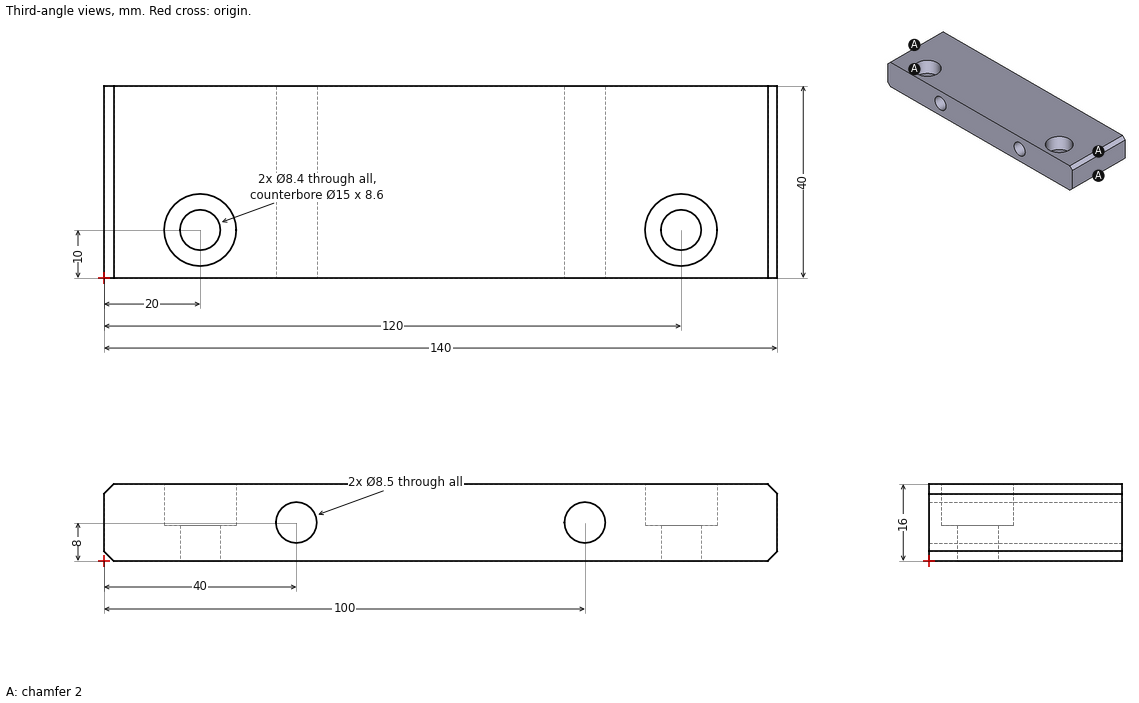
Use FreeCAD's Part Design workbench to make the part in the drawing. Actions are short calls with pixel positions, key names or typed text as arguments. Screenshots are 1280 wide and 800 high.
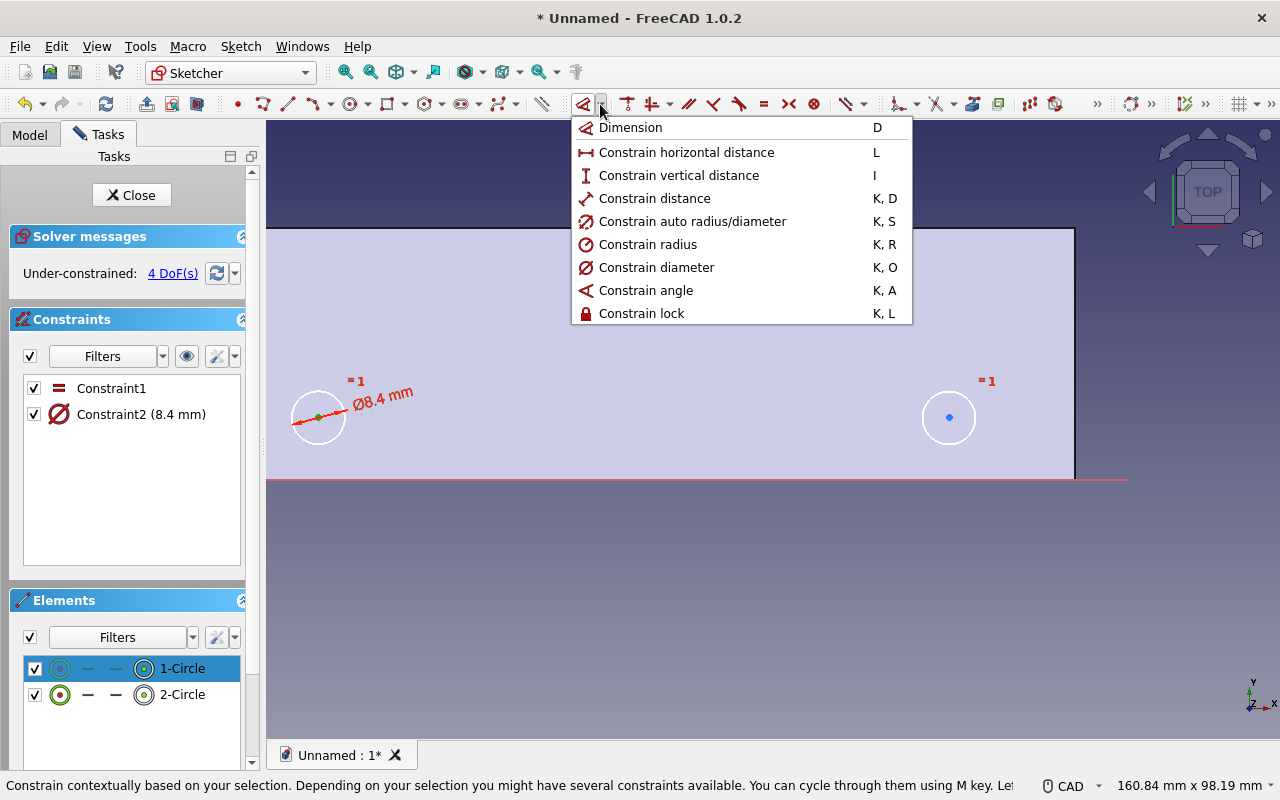
click(742, 152)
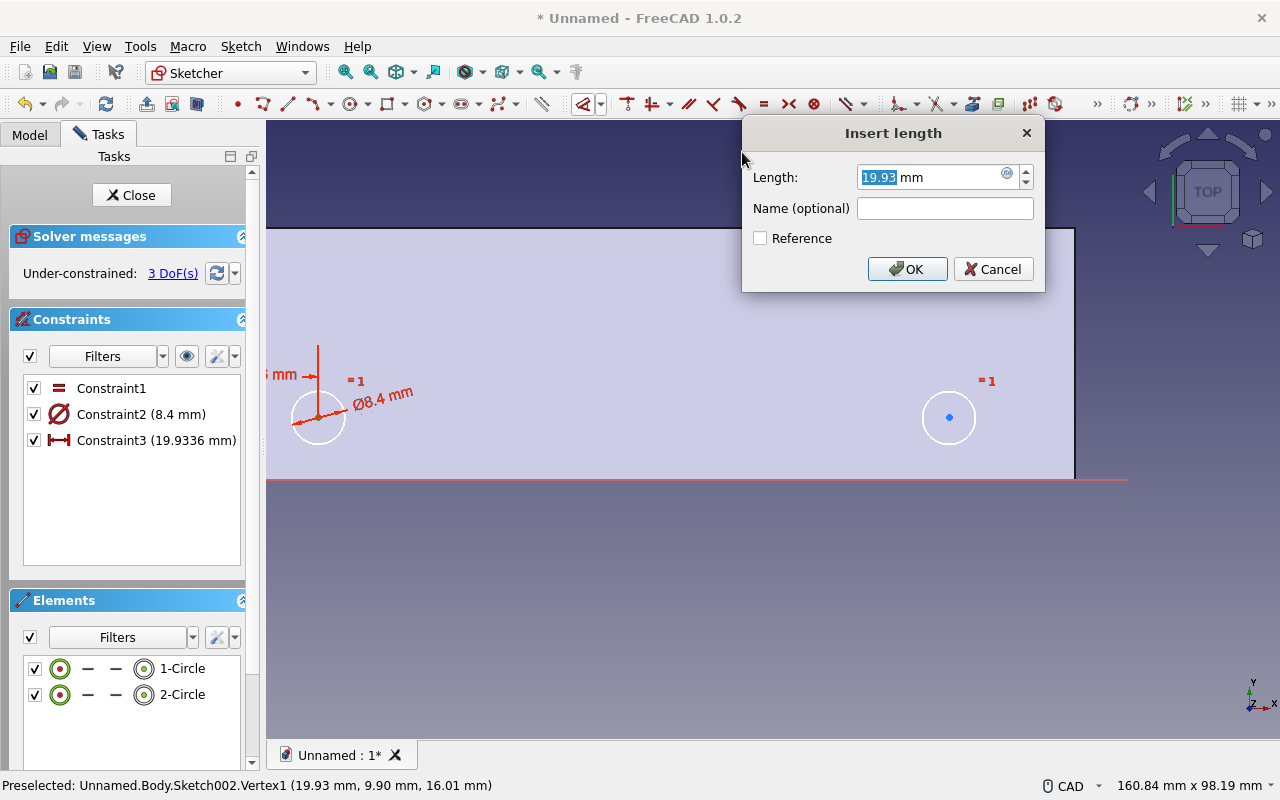
text(20)
key(Return)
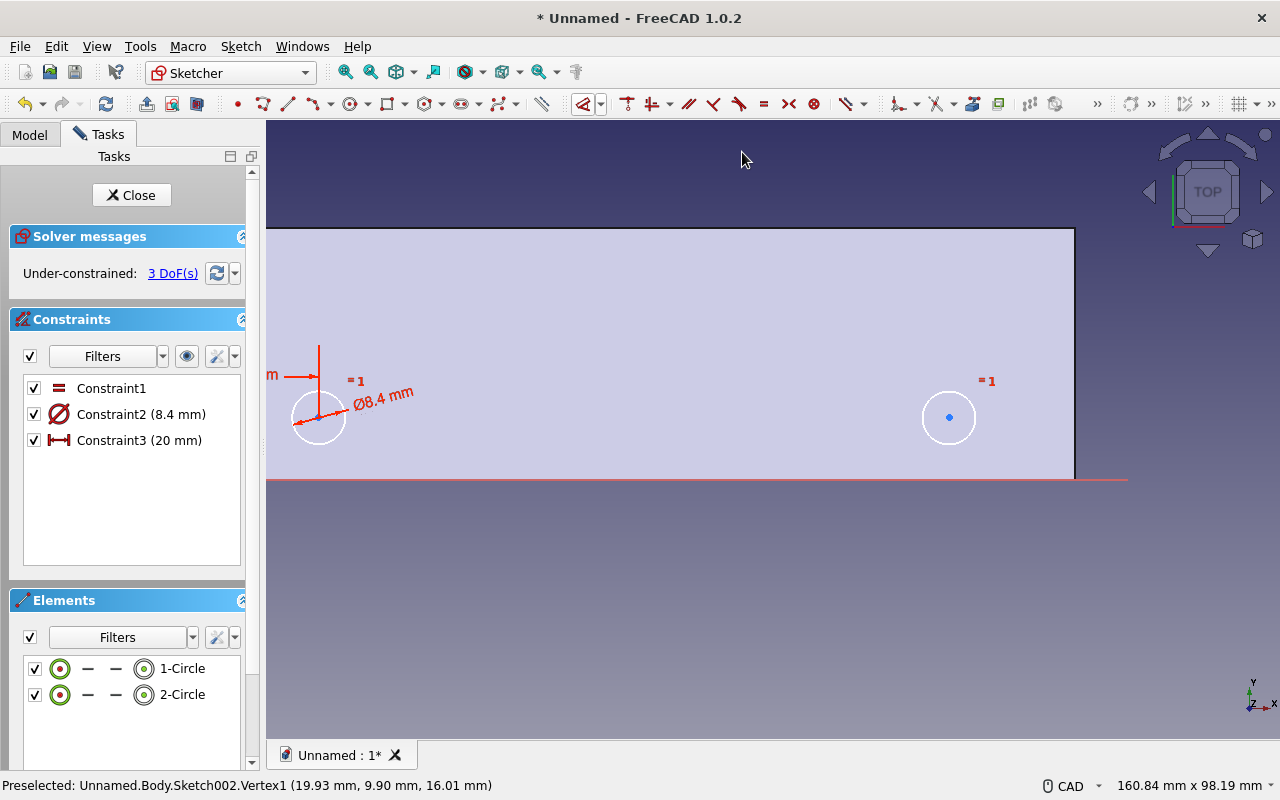
click(319, 418)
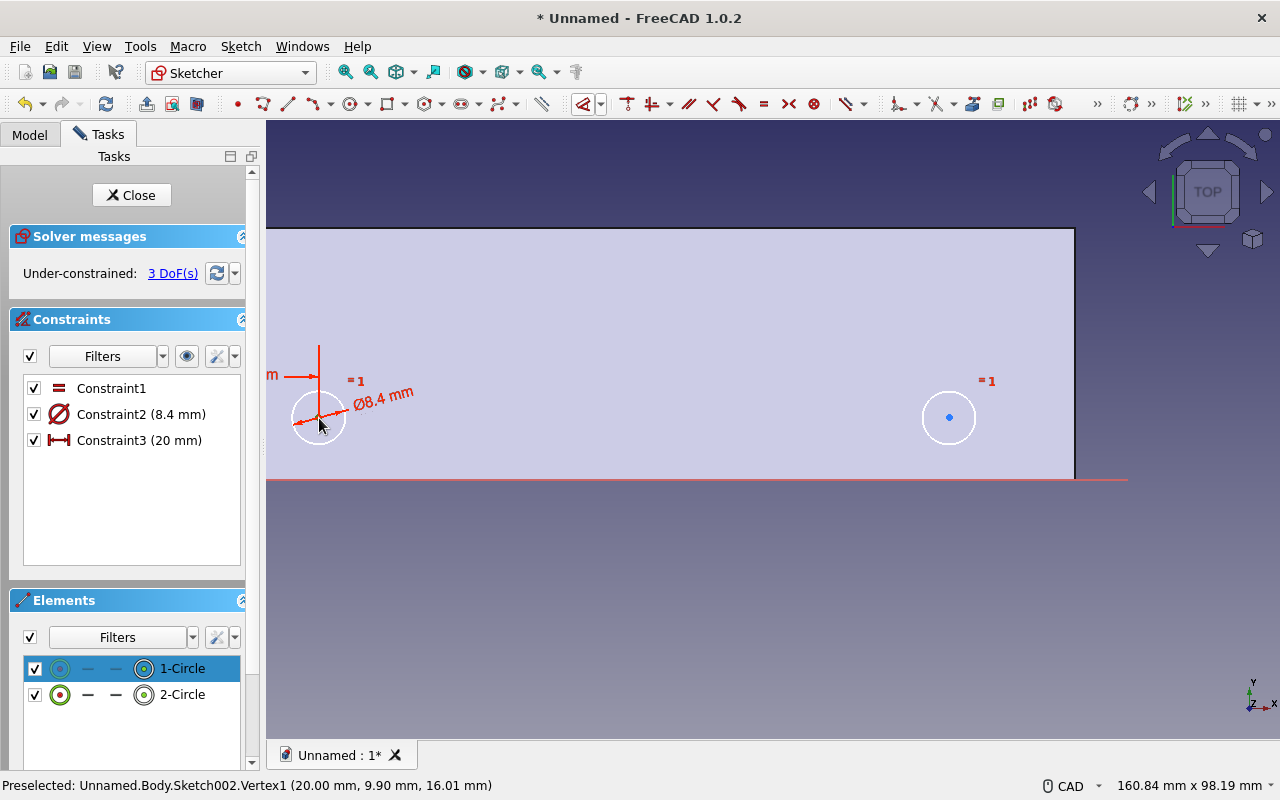
key(i)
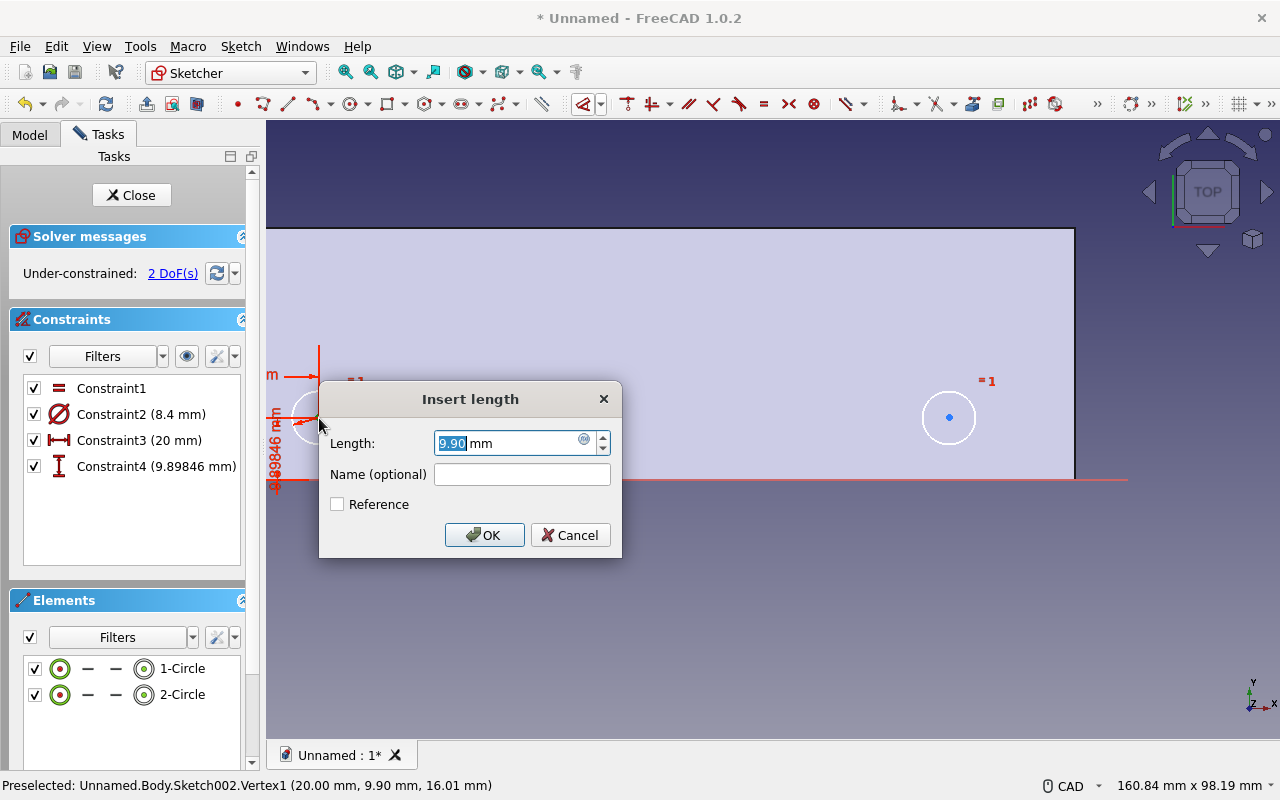
text(10)
key(Return)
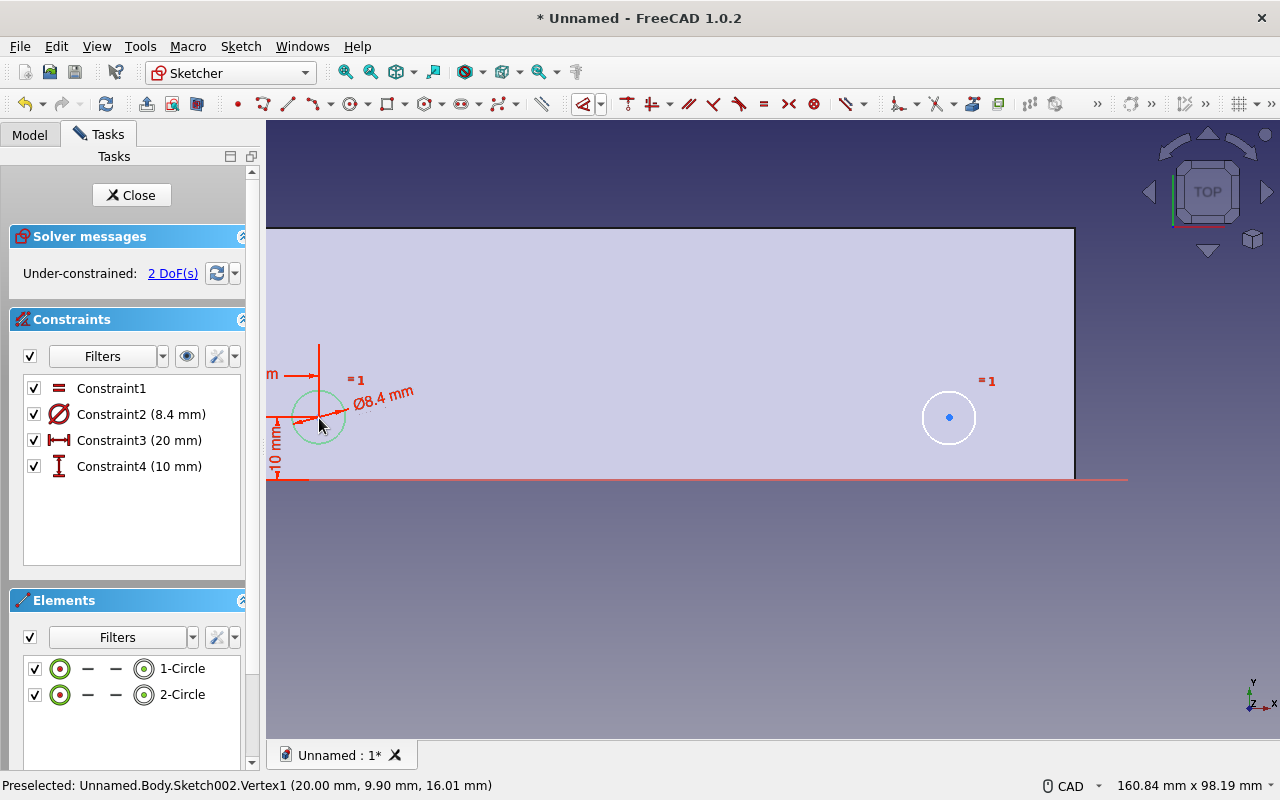
click(949, 418)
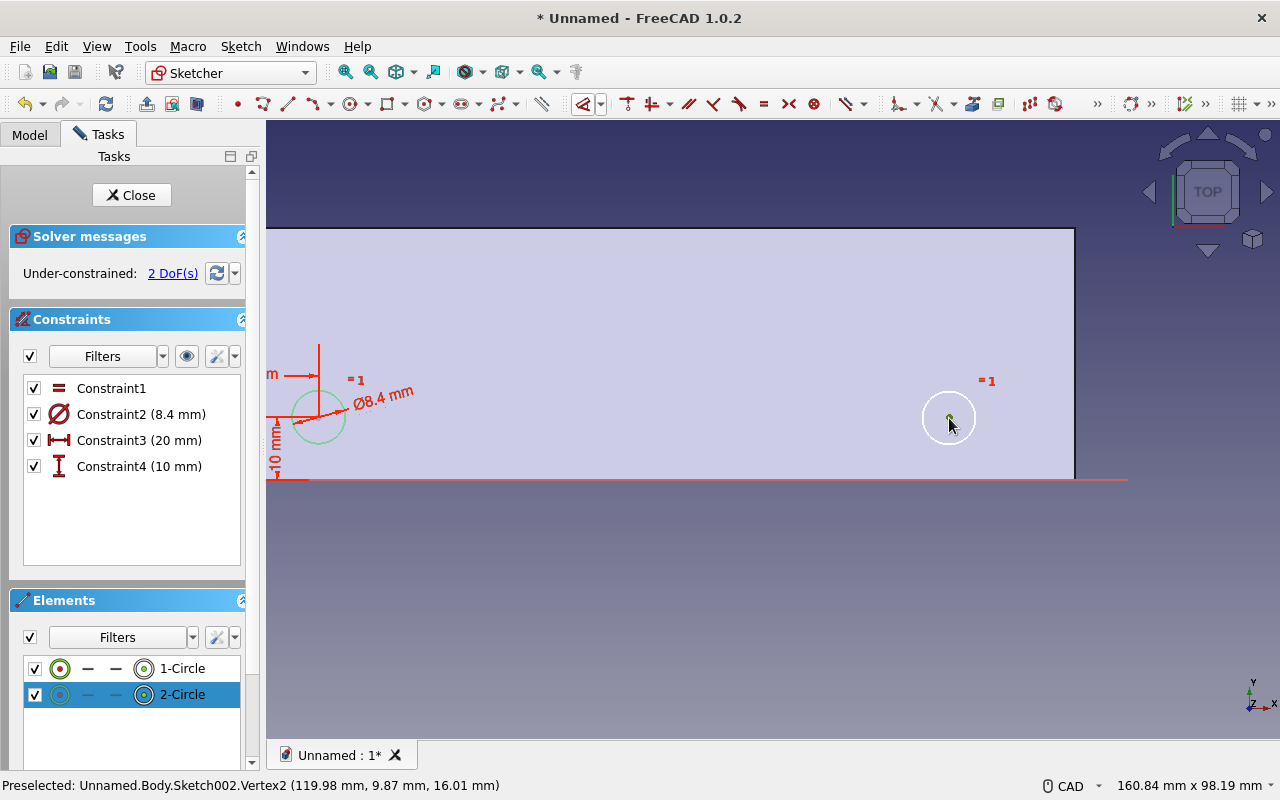
click(600, 104)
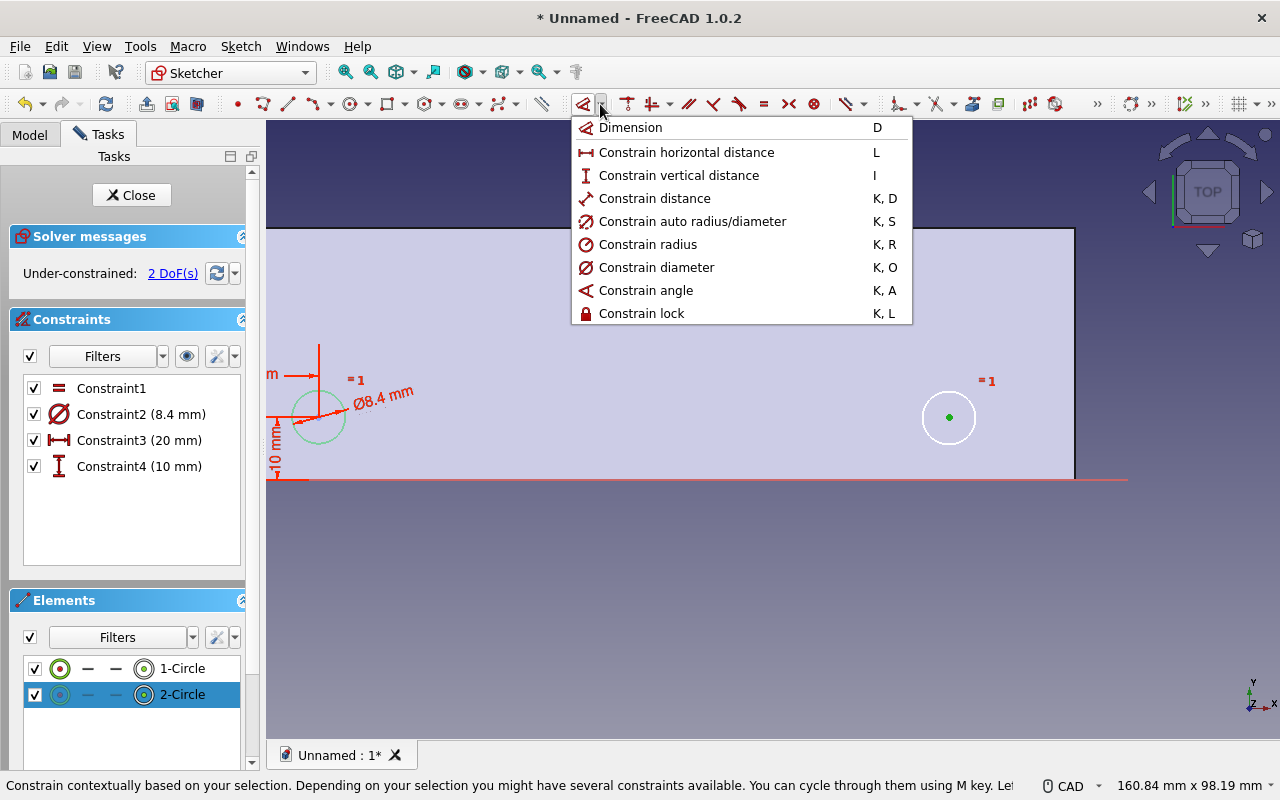
click(742, 176)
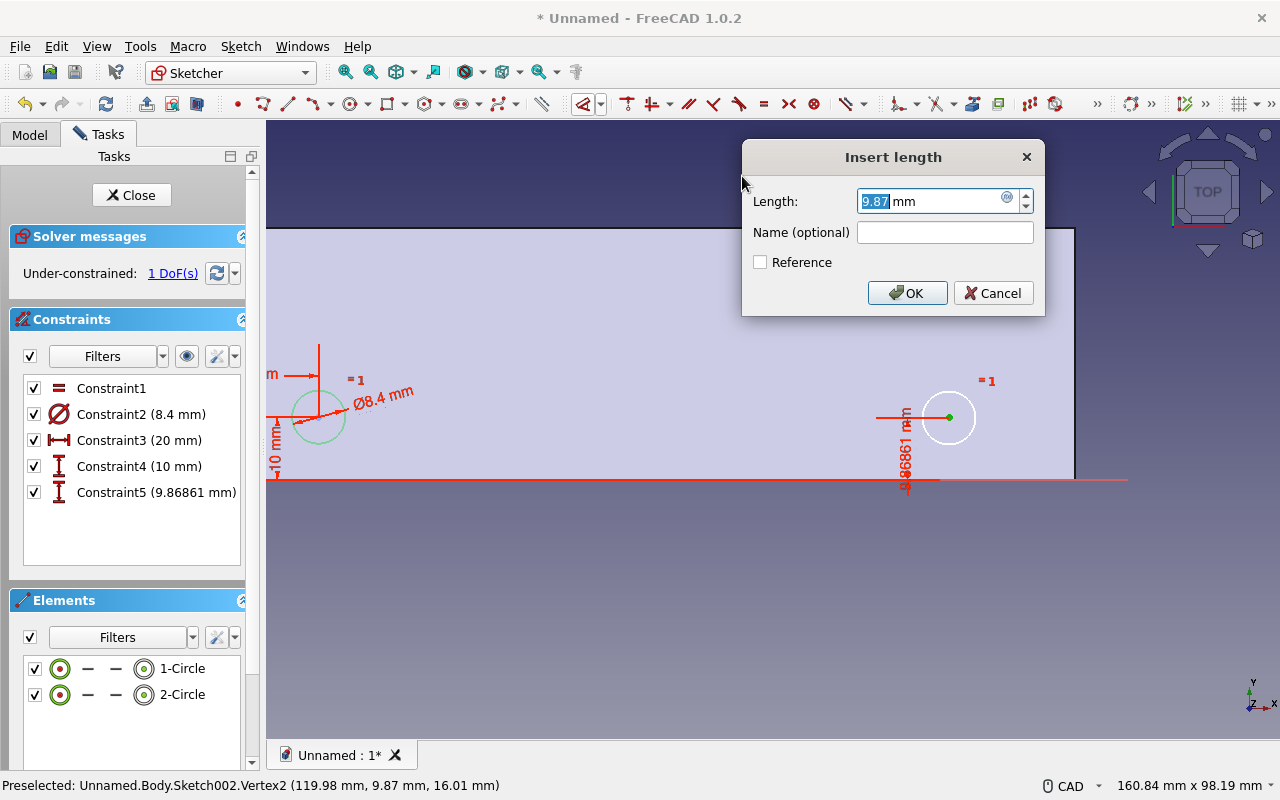
text(10)
key(Return)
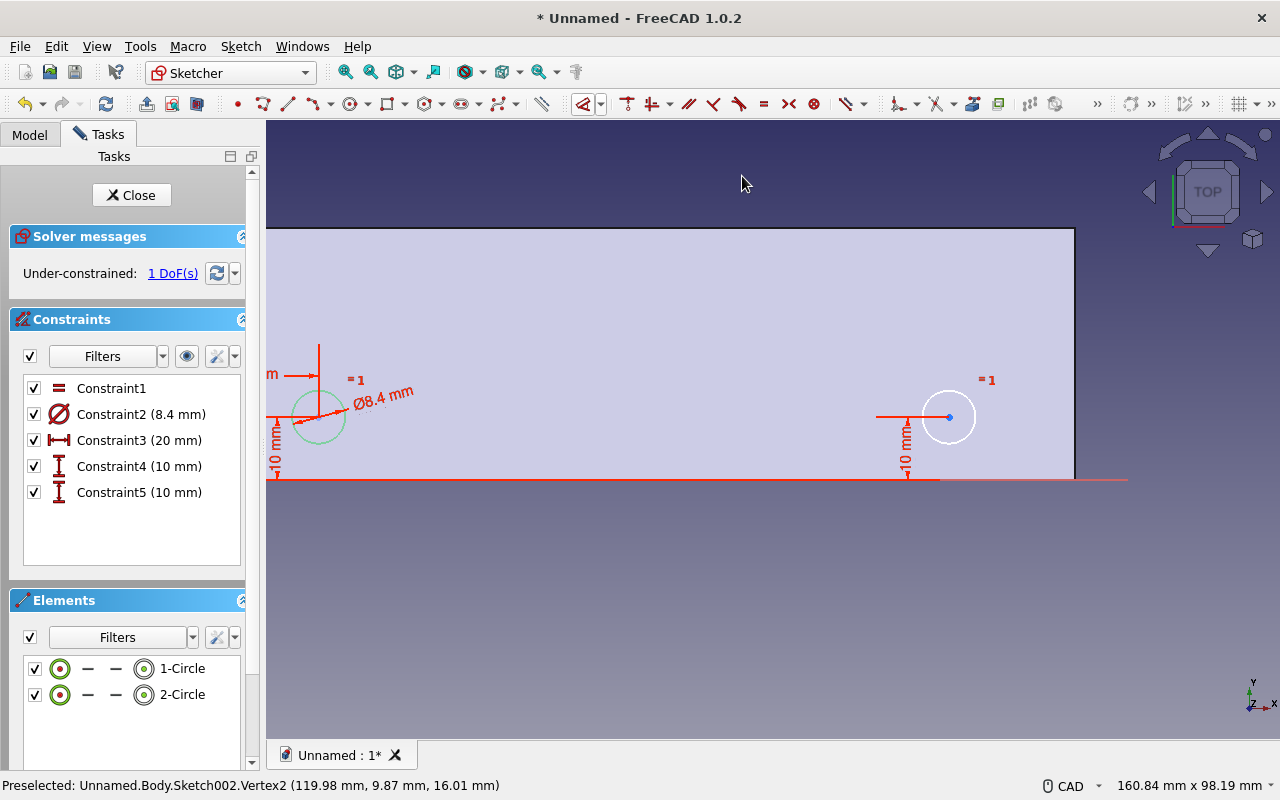
click(949, 417)